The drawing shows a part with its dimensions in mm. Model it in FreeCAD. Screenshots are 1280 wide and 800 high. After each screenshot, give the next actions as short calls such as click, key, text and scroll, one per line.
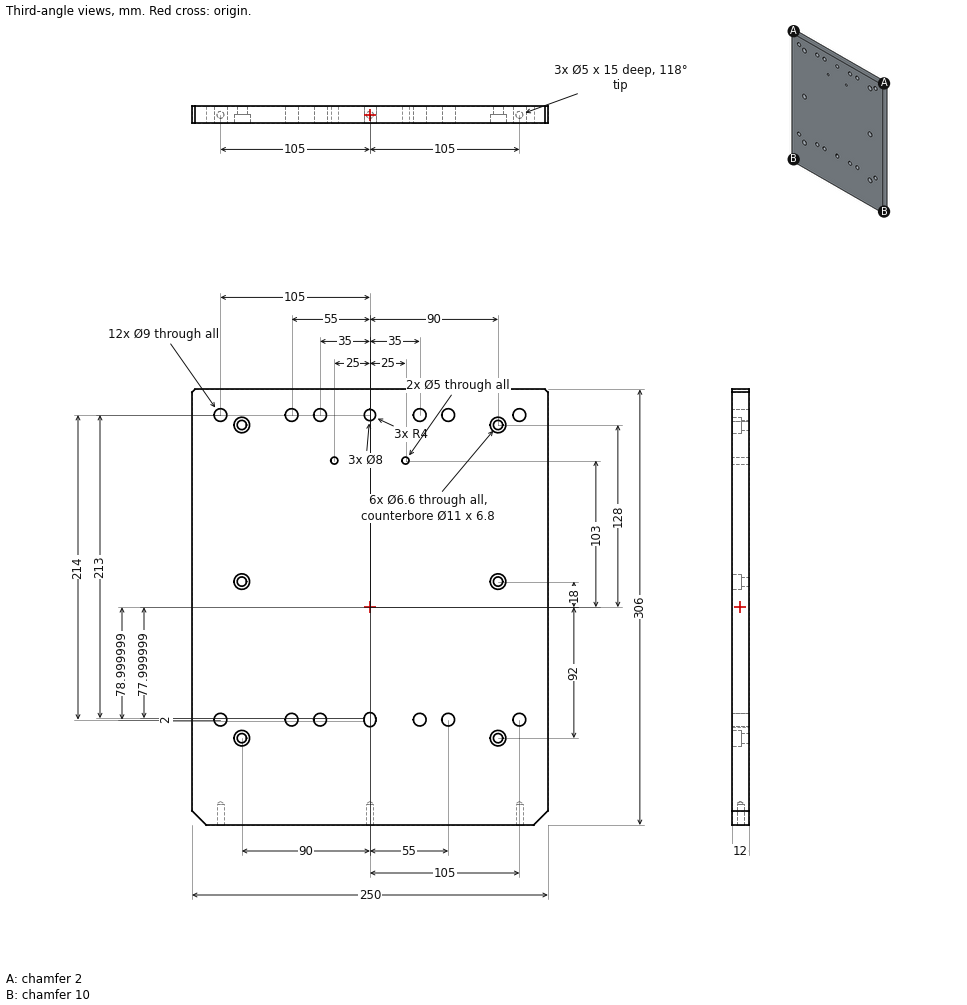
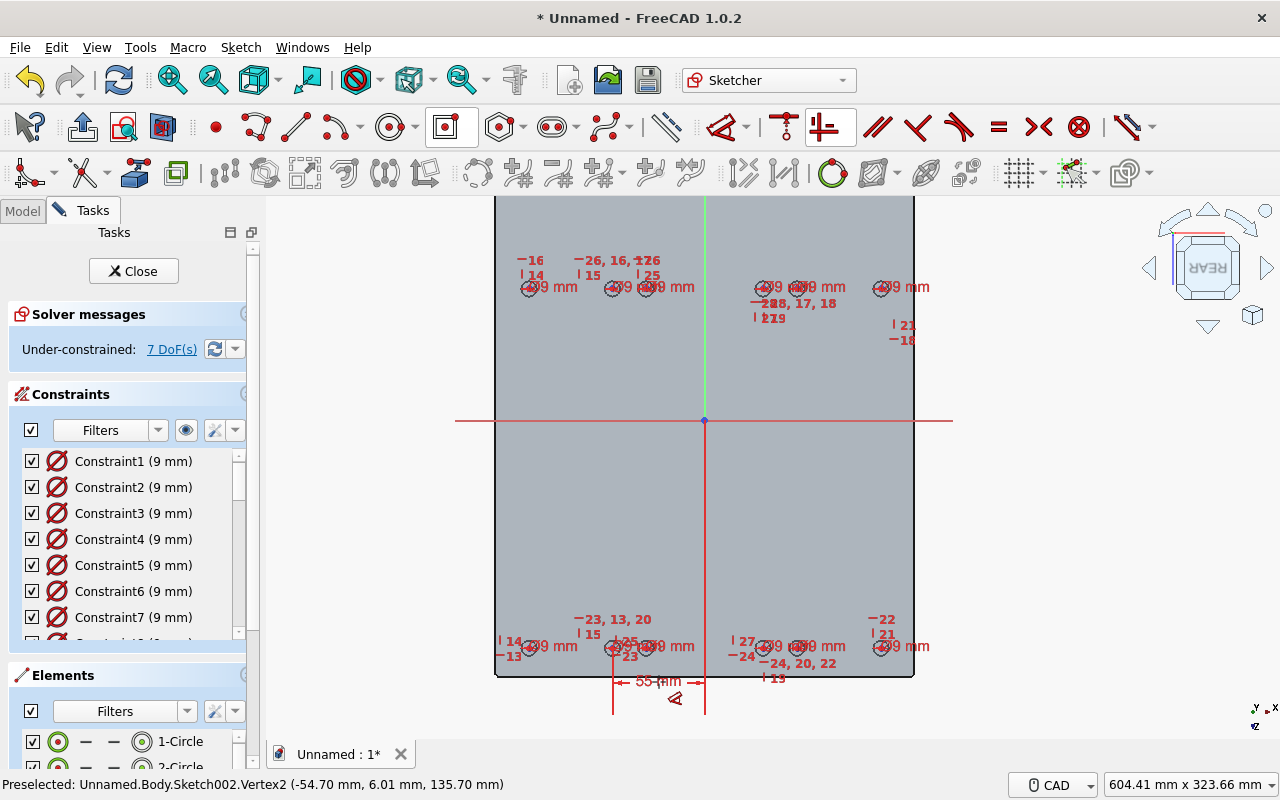
click(797, 289)
click(751, 255)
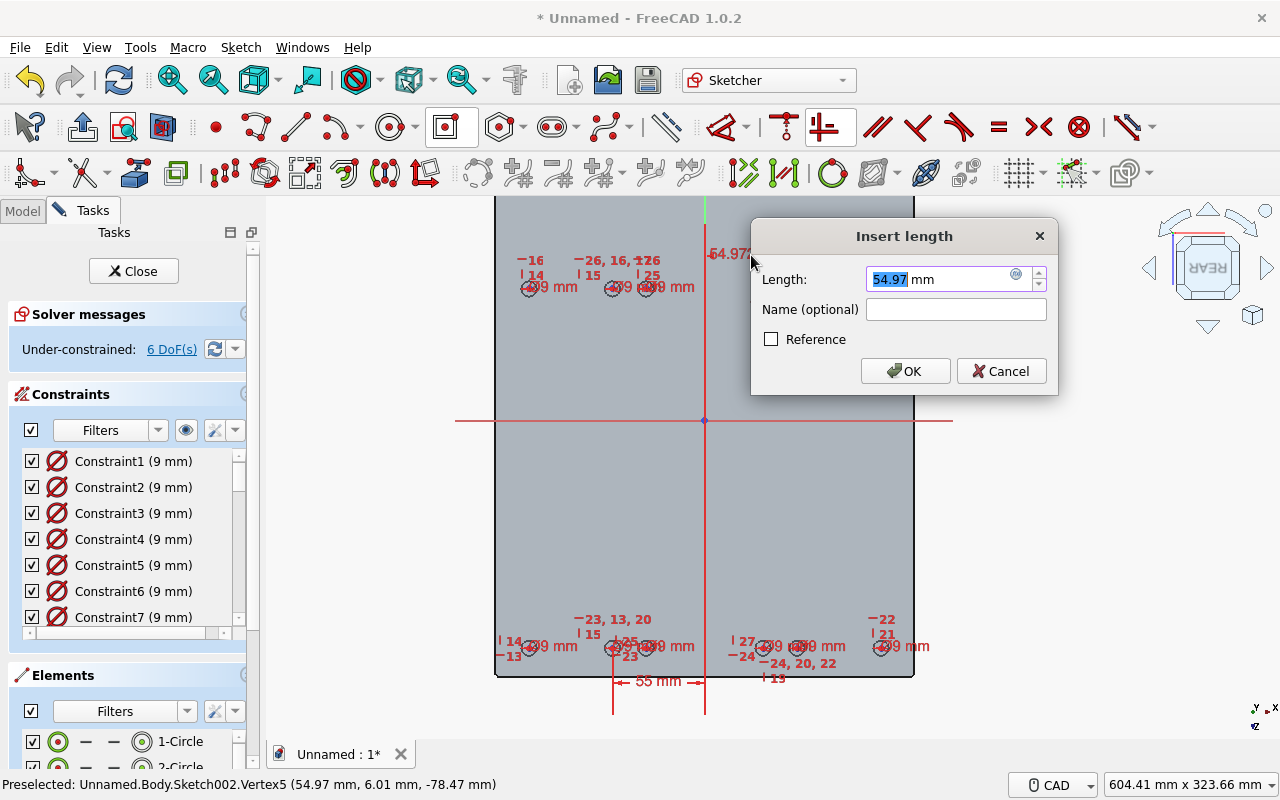
text(55)
key(Return)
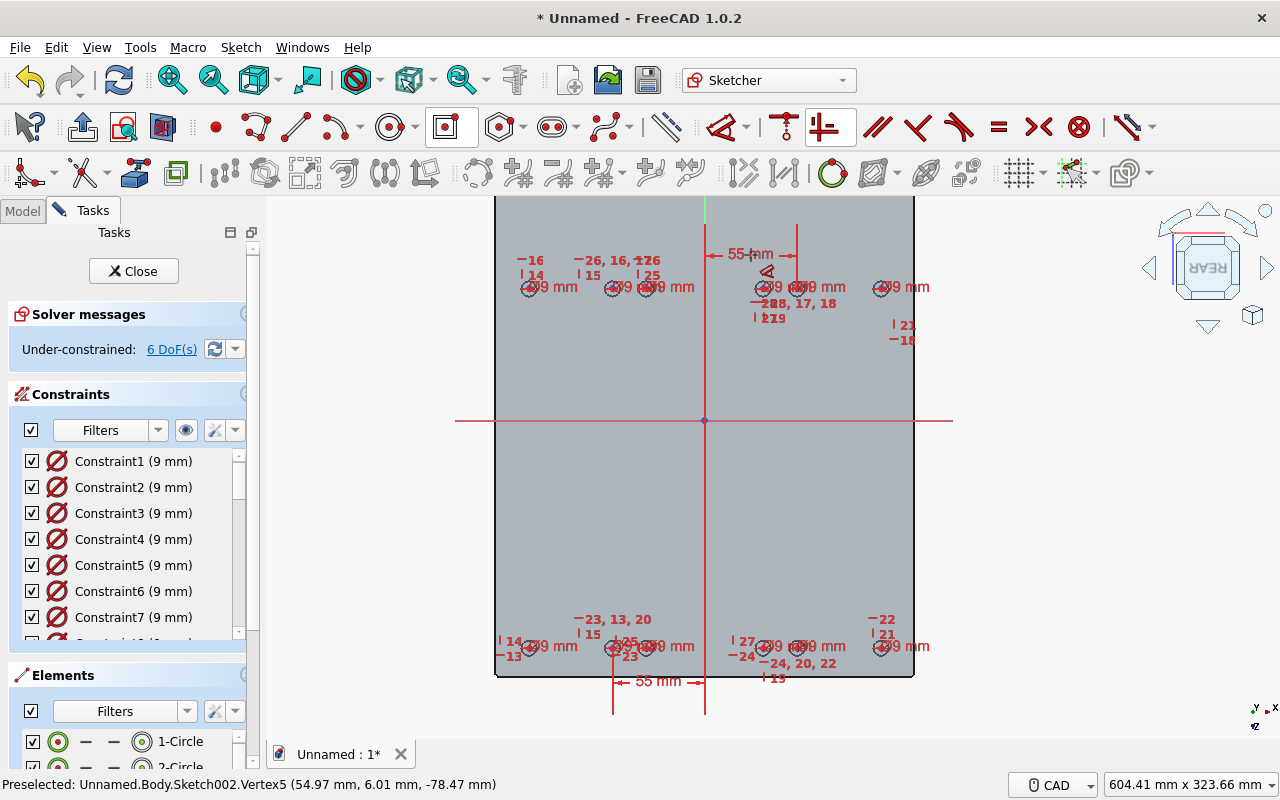
click(646, 648)
click(675, 387)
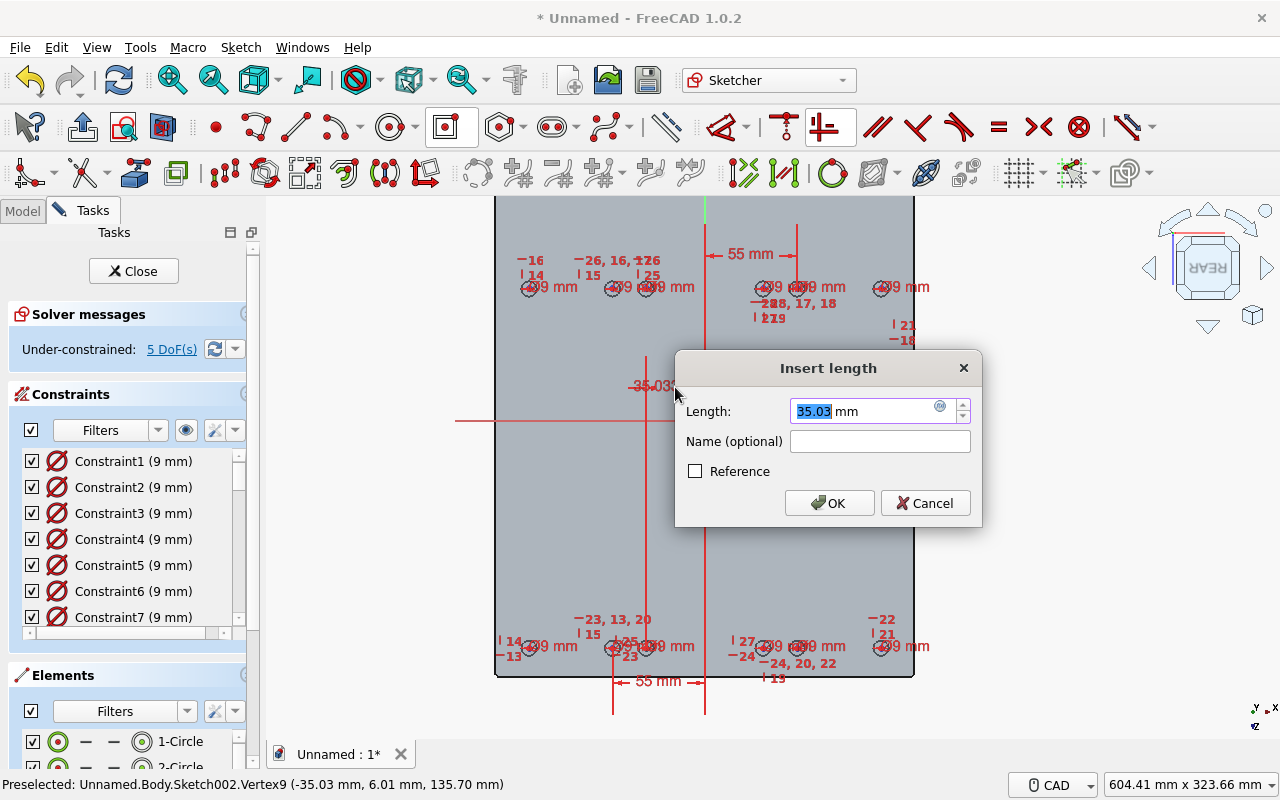
text(35)
key(Return)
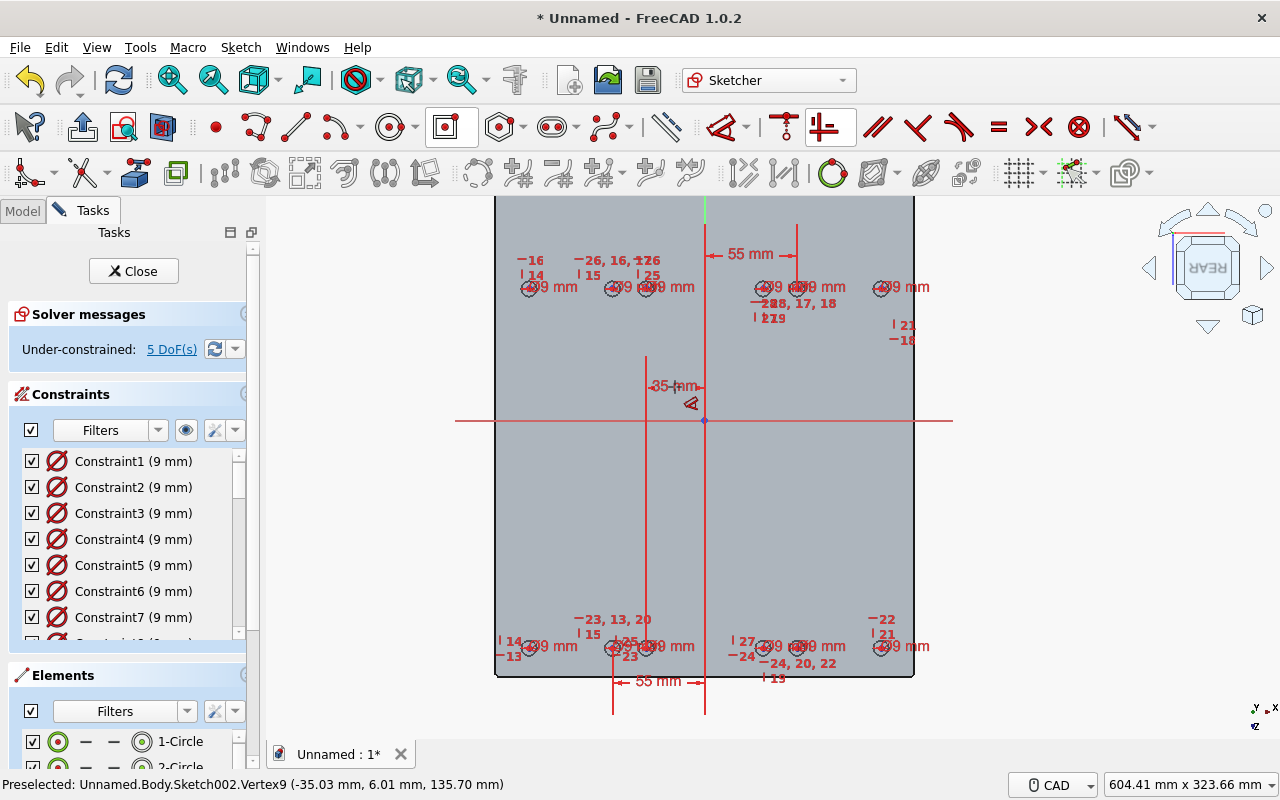
click(763, 648)
click(734, 682)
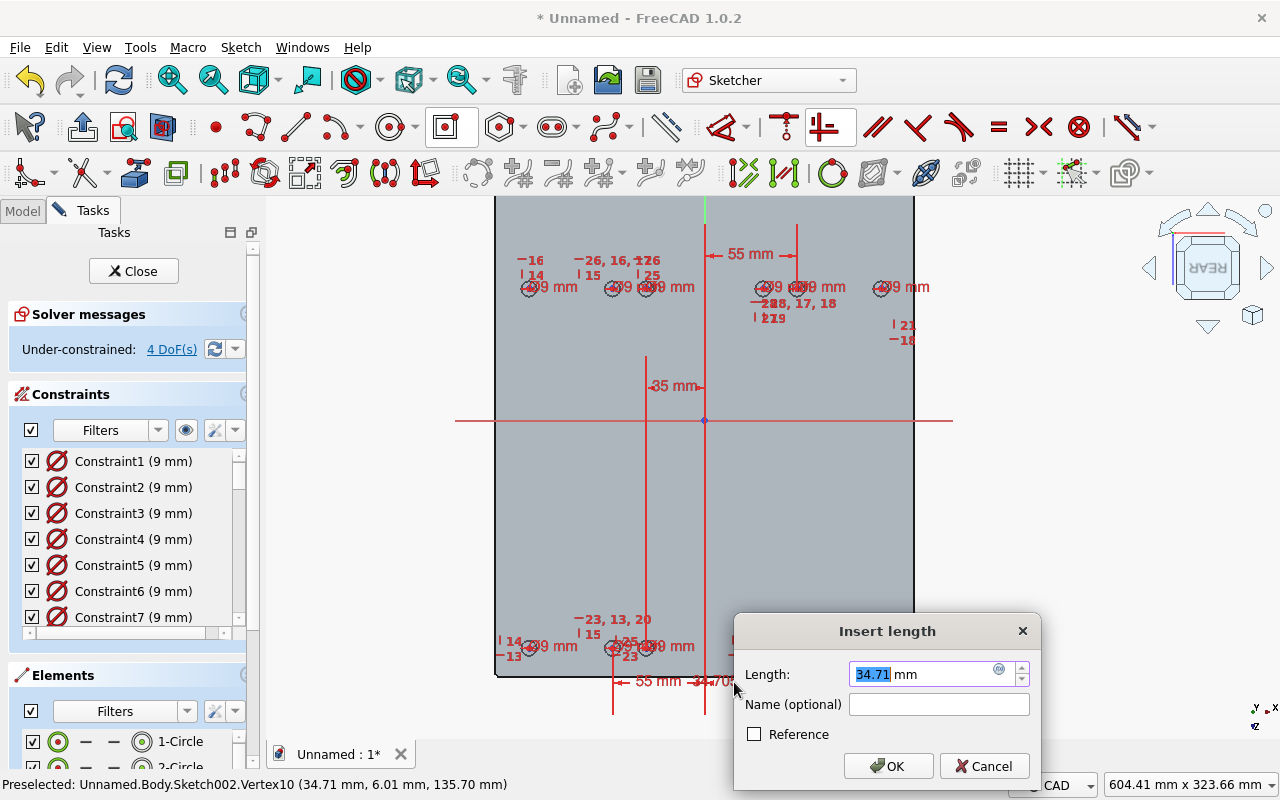
text(35)
key(Return)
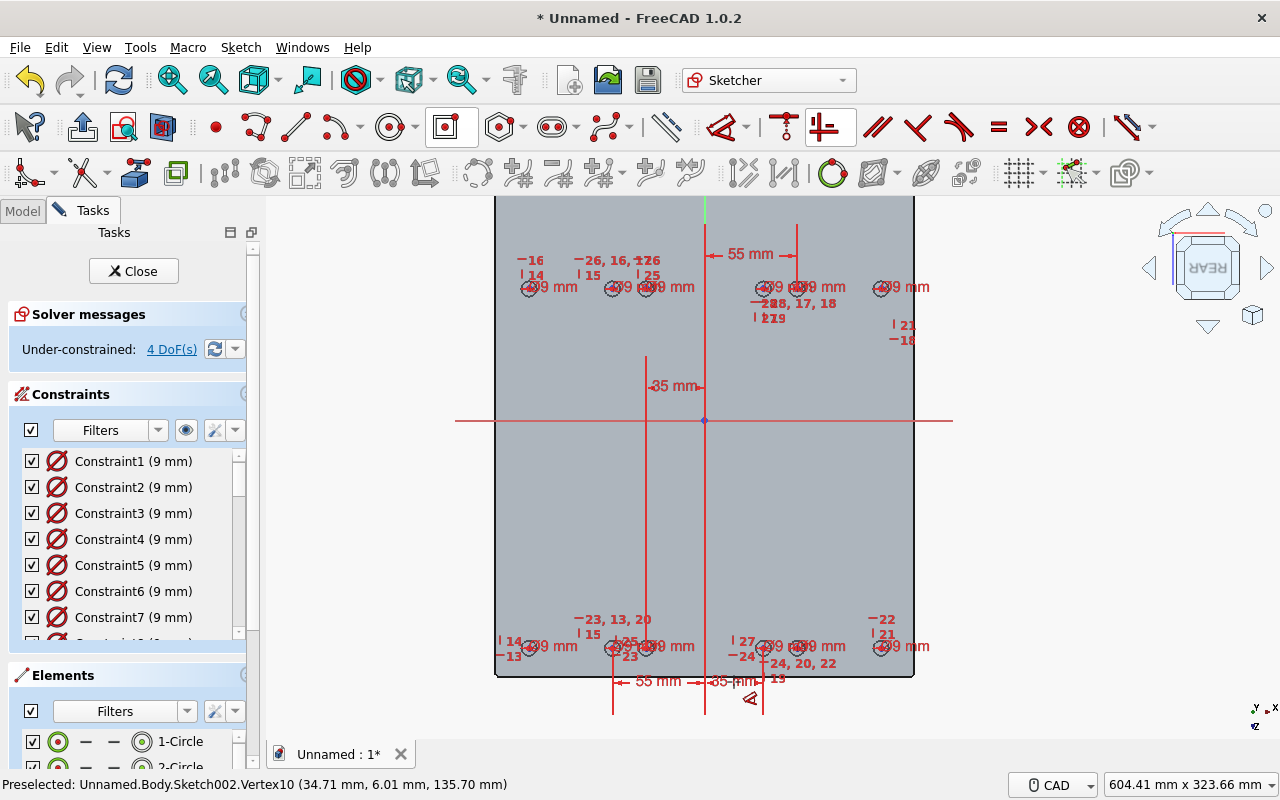
click(529, 648)
click(576, 682)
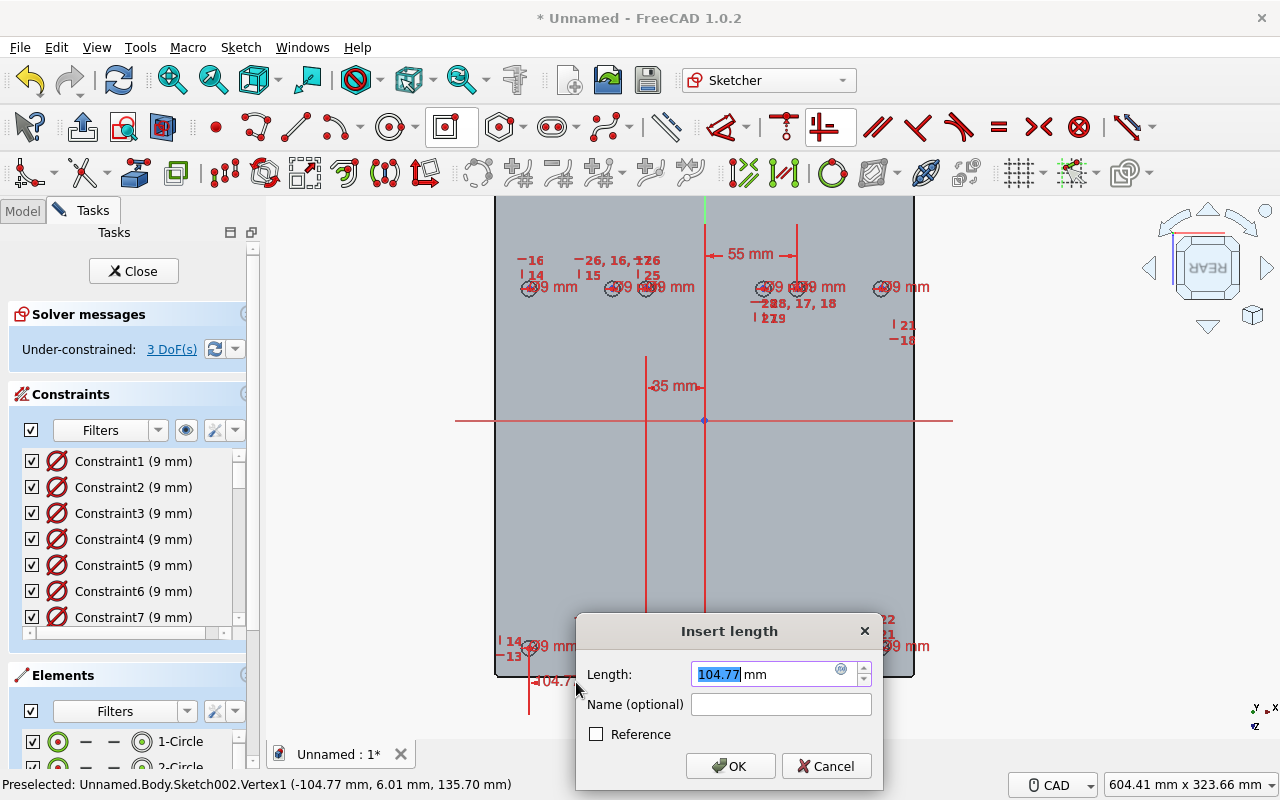
text(105)
key(Return)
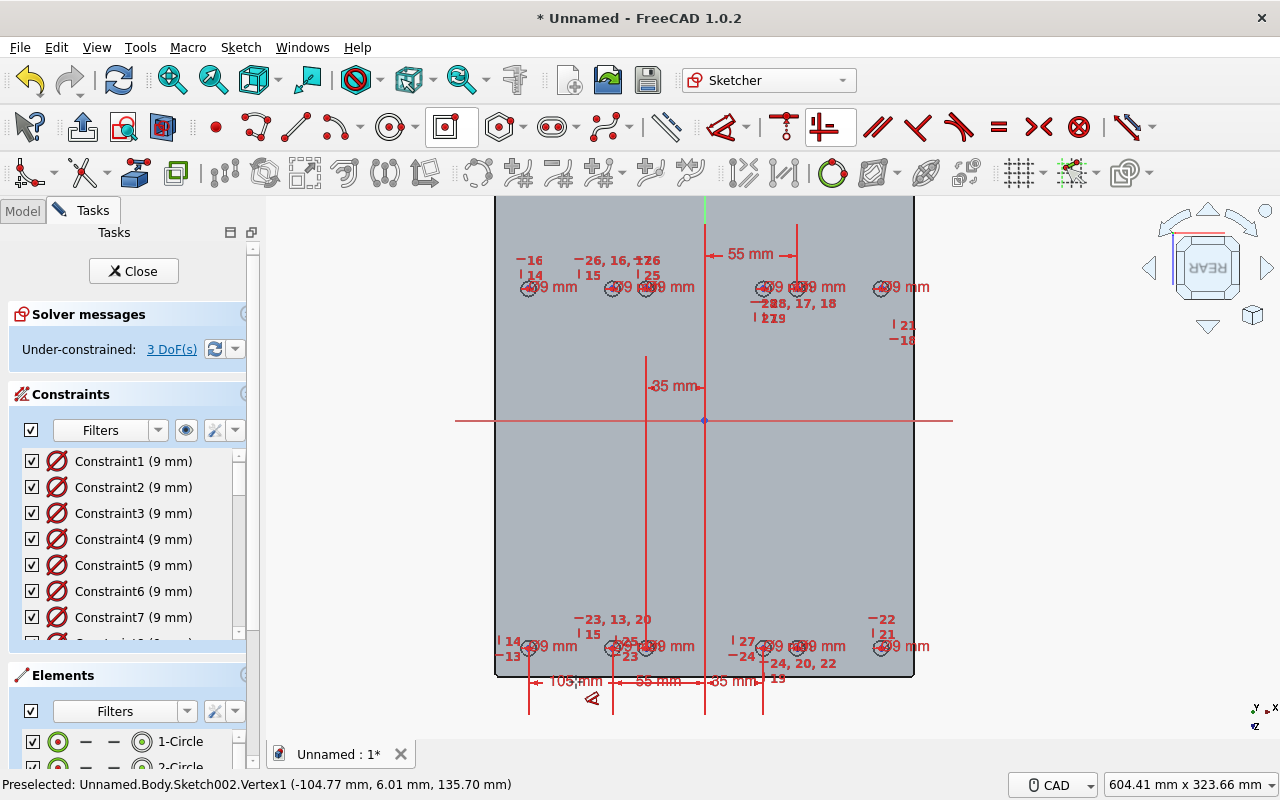
click(881, 289)
click(833, 255)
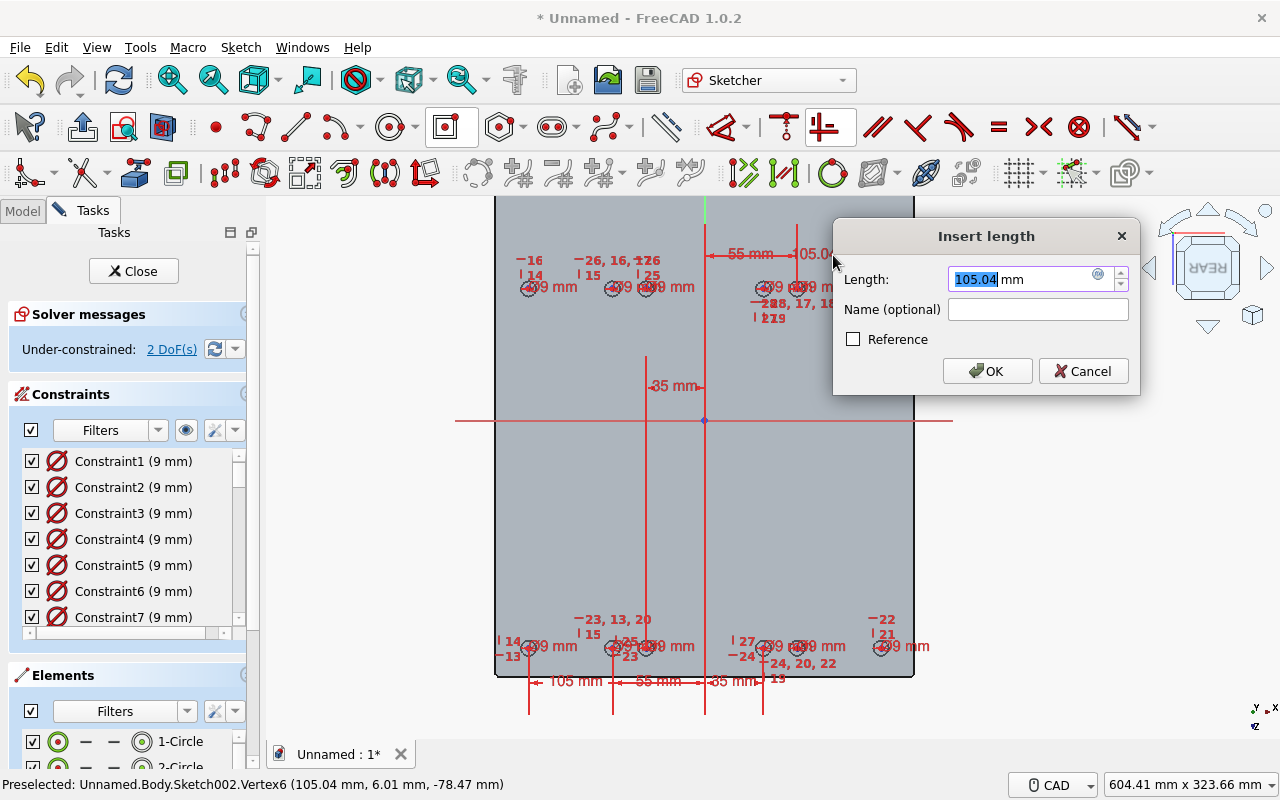
text(105)
key(Return)